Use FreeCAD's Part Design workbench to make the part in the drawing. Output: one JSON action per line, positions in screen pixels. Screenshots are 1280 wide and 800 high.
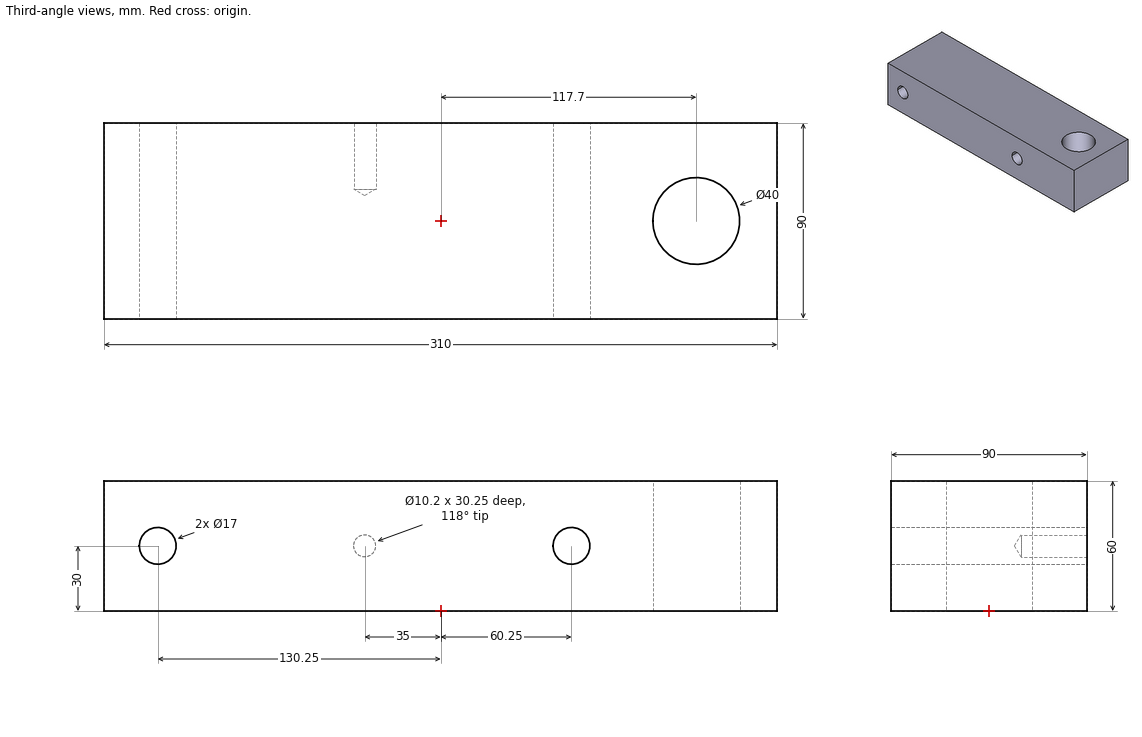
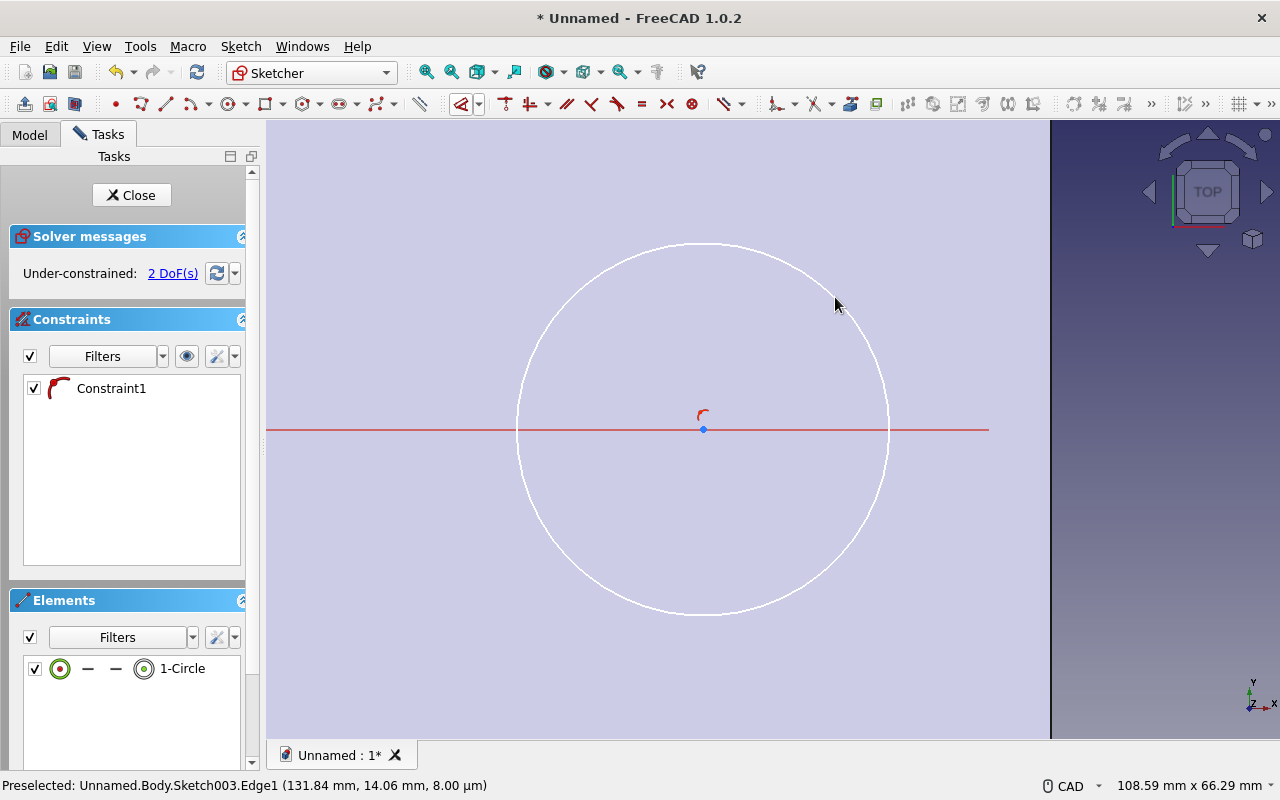
{"action": "left_click", "coordinate": [834, 297]}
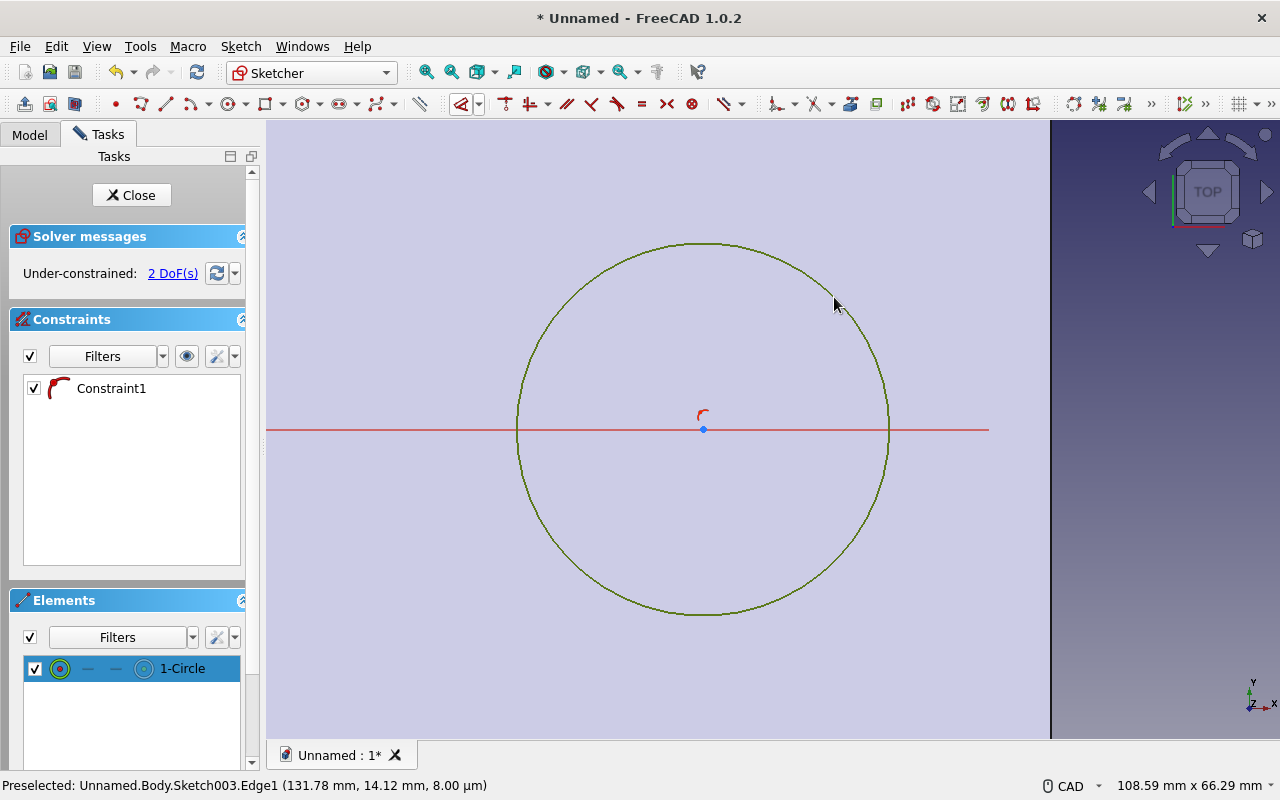
{"action": "key", "text": "k o"}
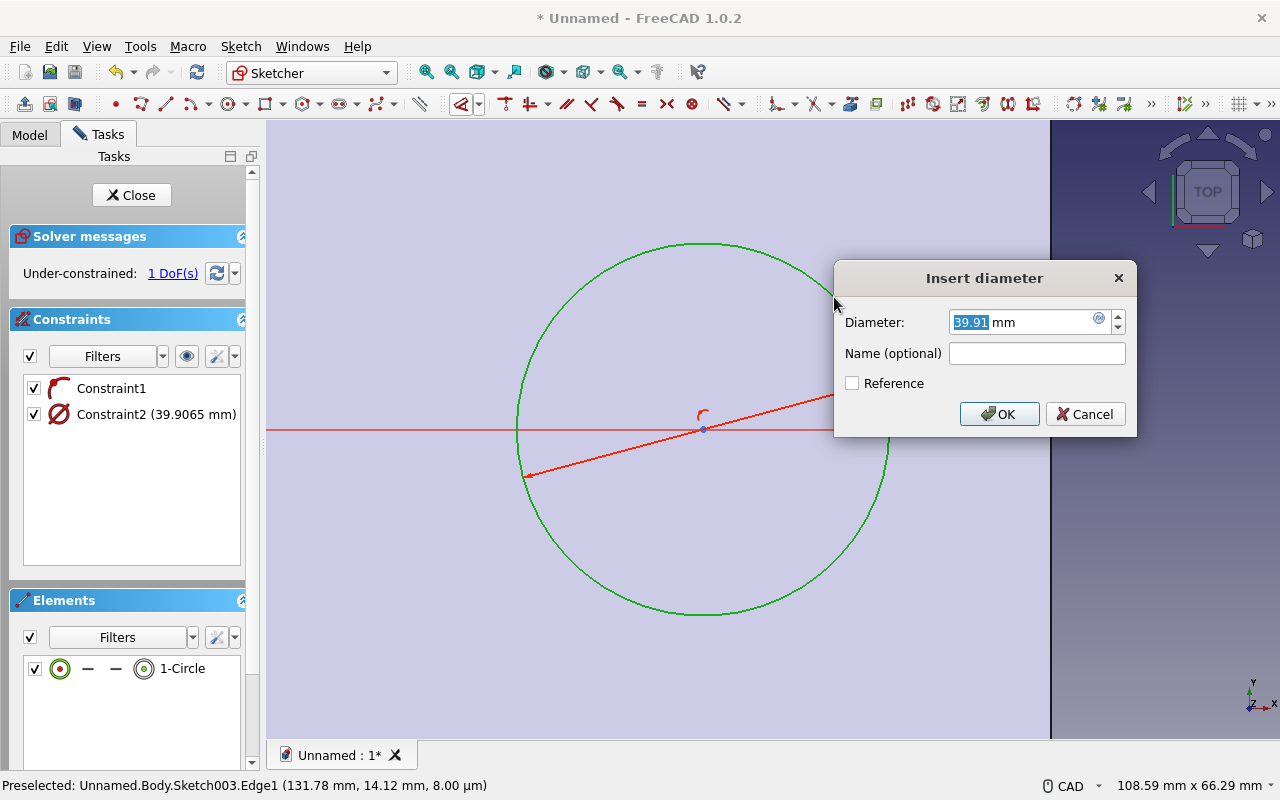
{"action": "type", "text": "40"}
{"action": "key", "text": "Return"}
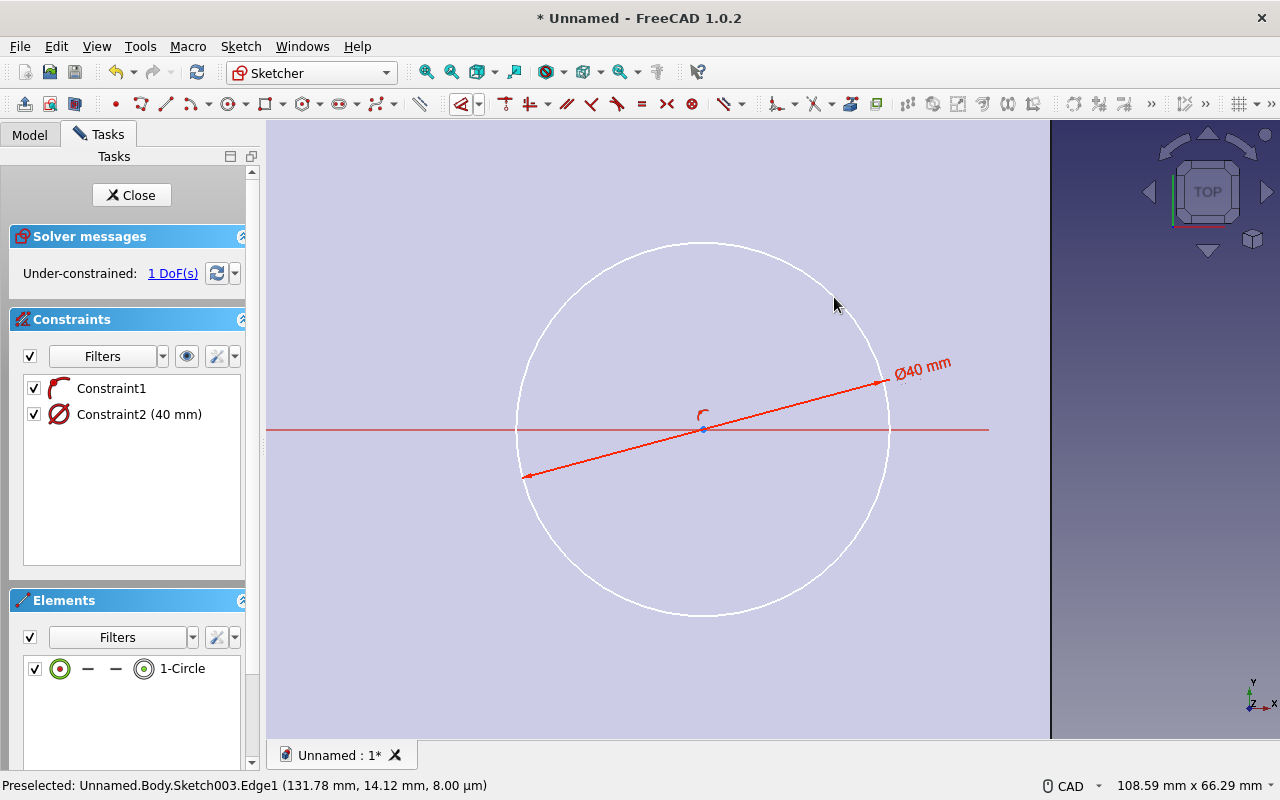
{"action": "left_click", "coordinate": [703, 429]}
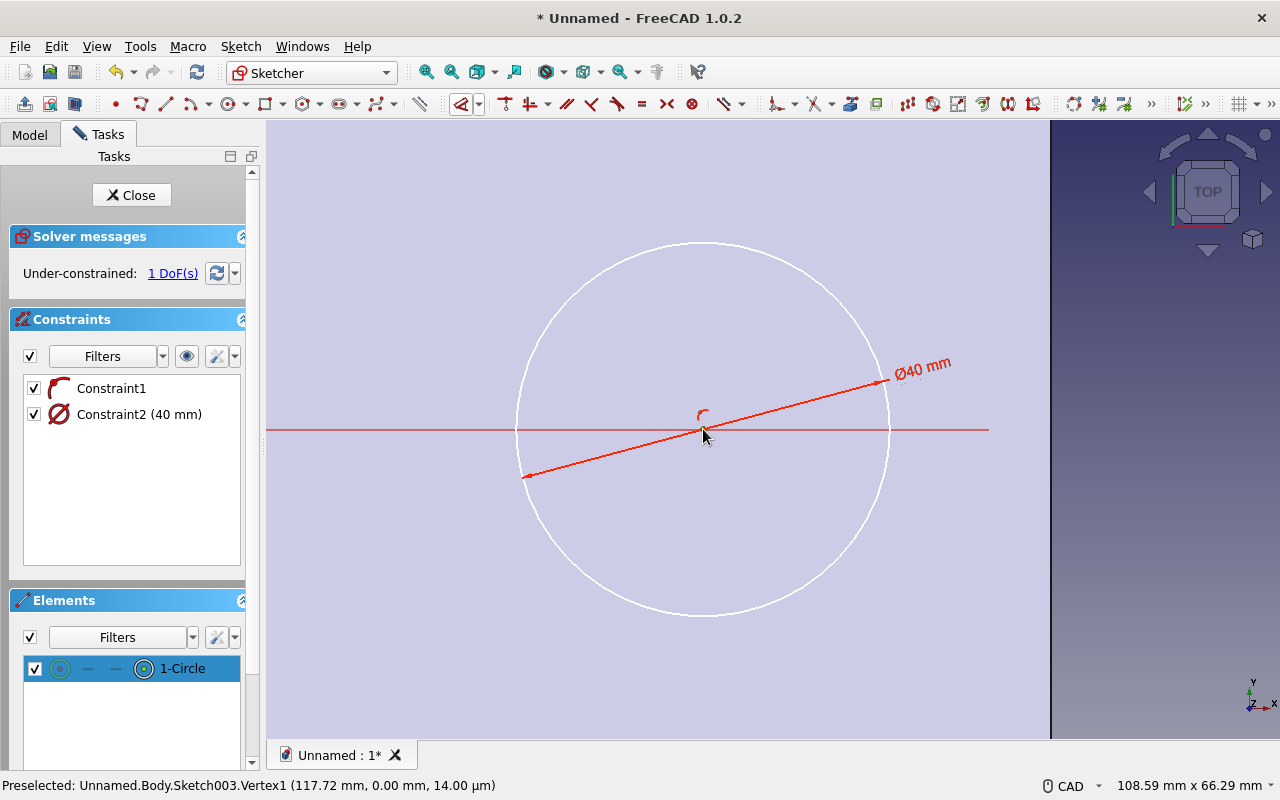
{"action": "left_click", "coordinate": [478, 104]}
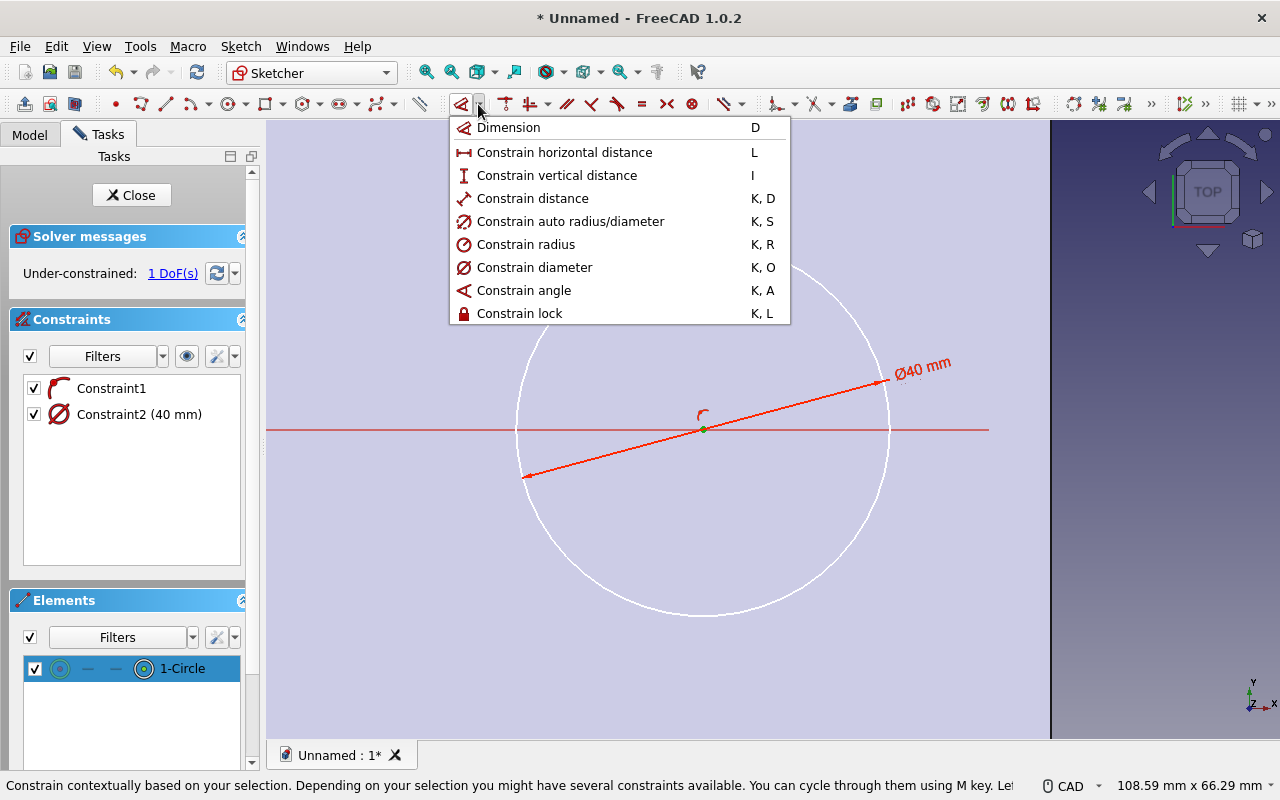
{"action": "left_click", "coordinate": [620, 152]}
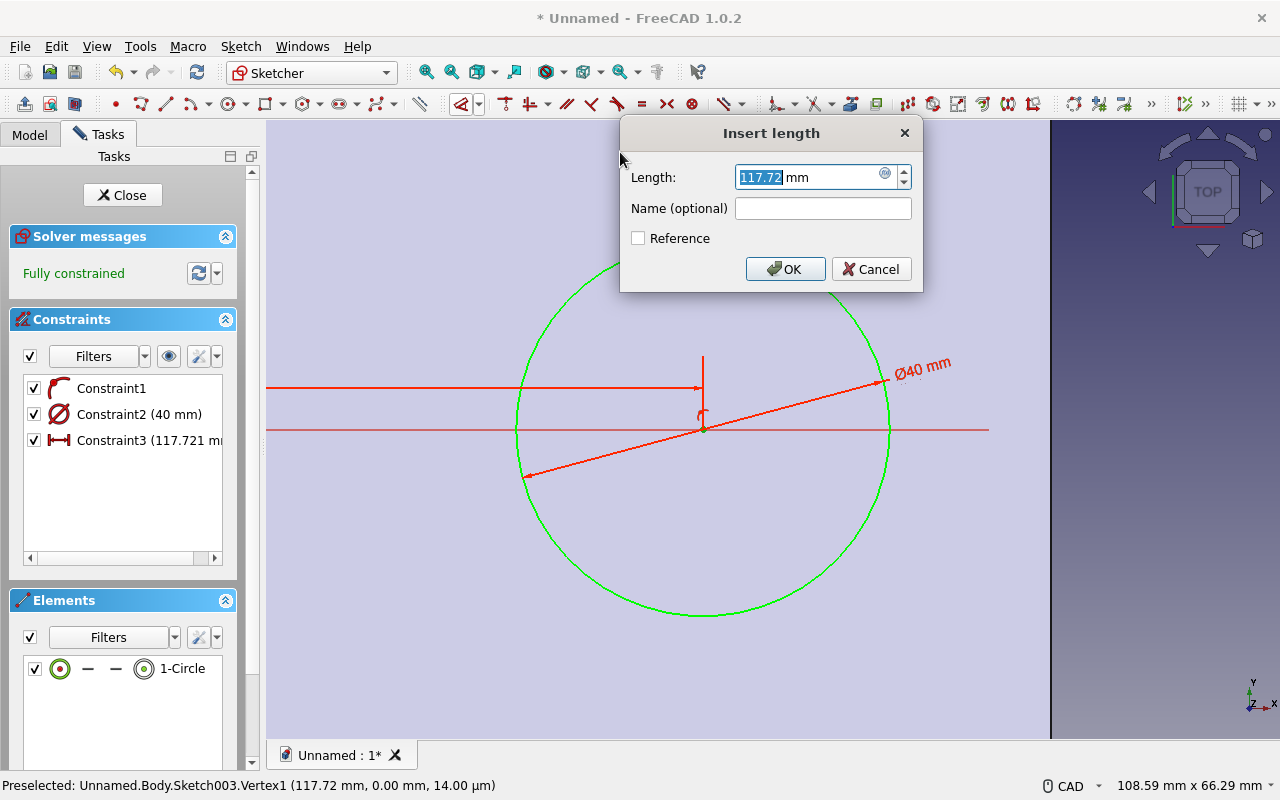
{"action": "type", "text": "117.7"}
{"action": "key", "text": "Return"}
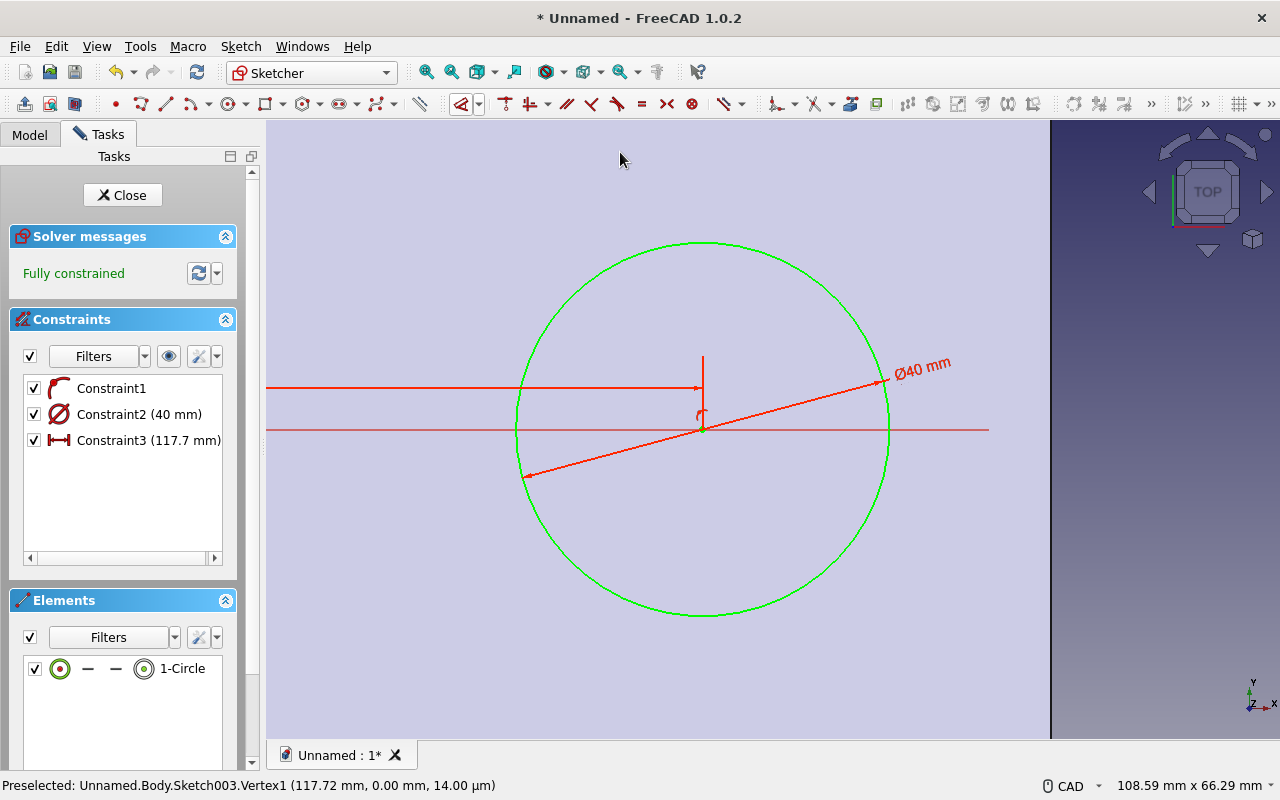
{"action": "left_click", "coordinate": [123, 195]}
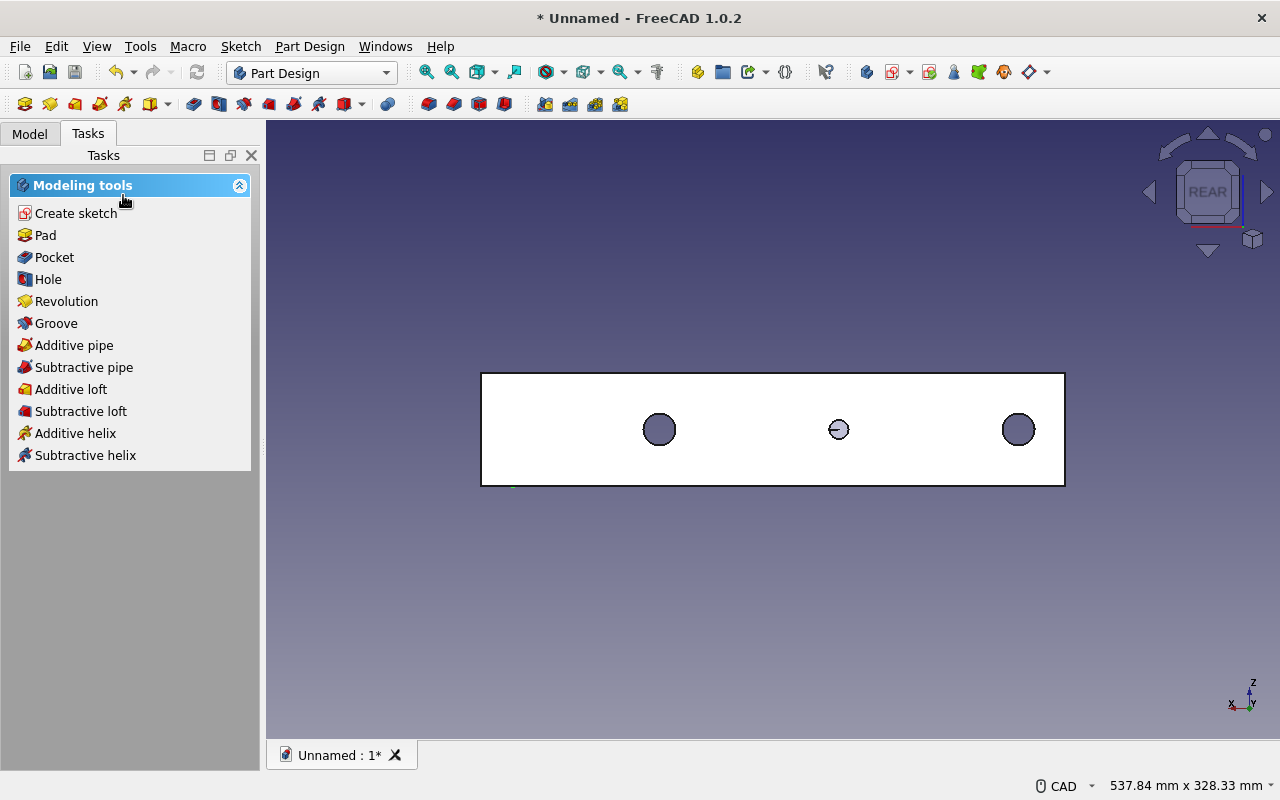
{"action": "left_click", "coordinate": [194, 104]}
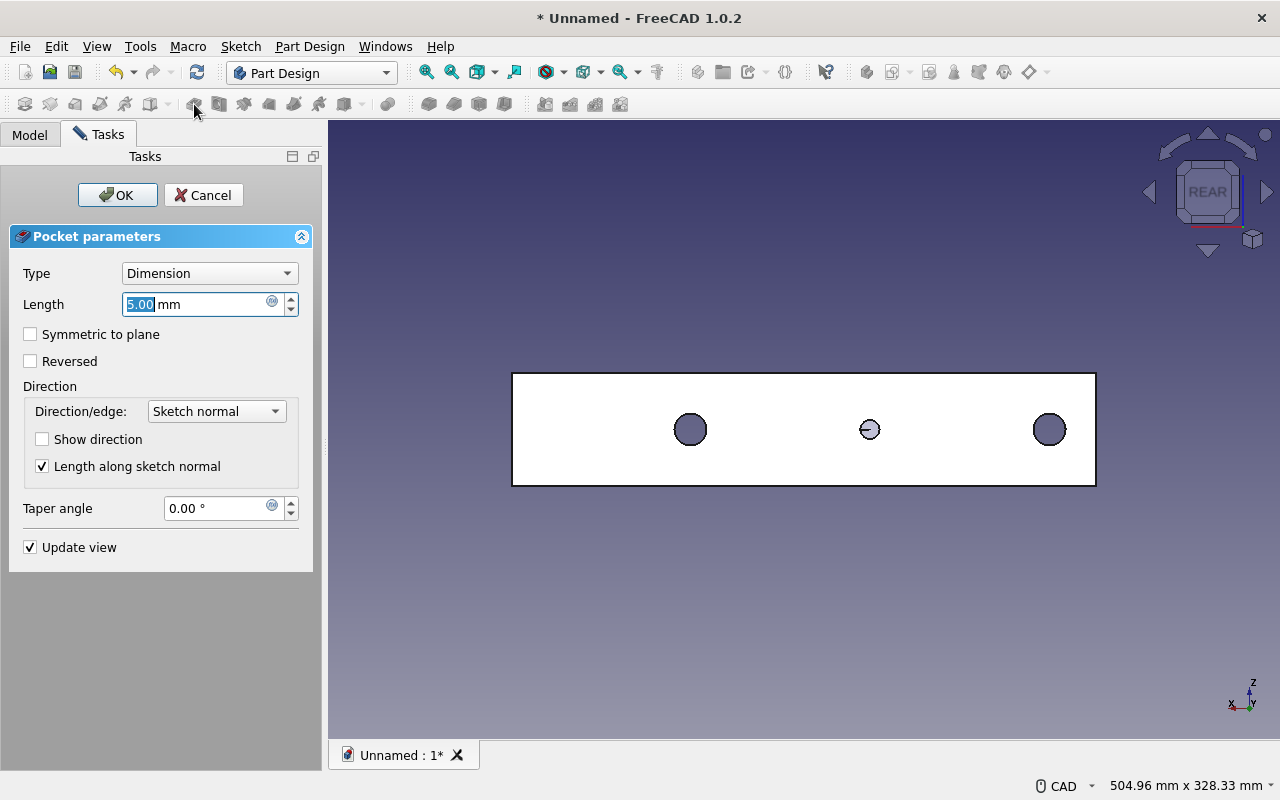
{"action": "type", "text": "60"}
{"action": "key", "text": "Tab"}